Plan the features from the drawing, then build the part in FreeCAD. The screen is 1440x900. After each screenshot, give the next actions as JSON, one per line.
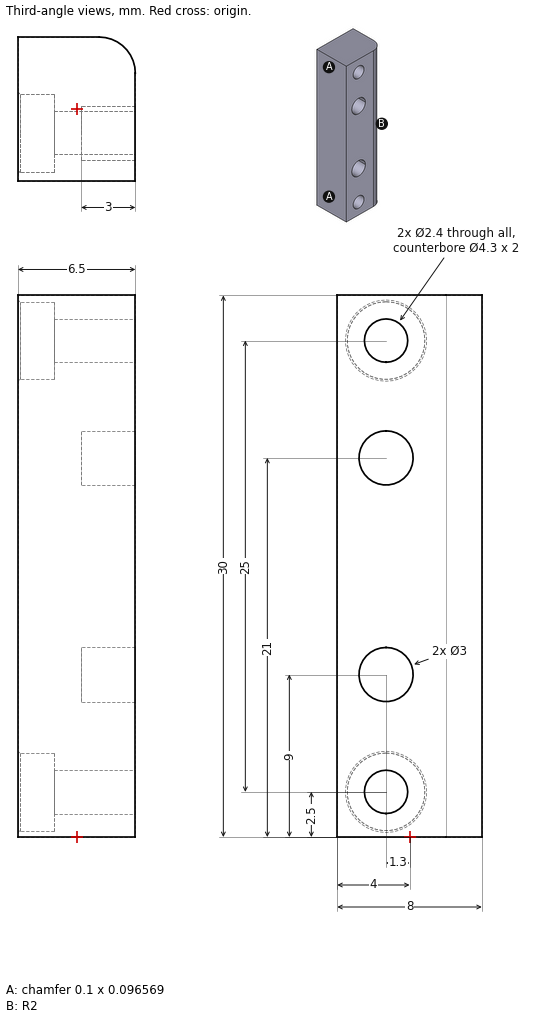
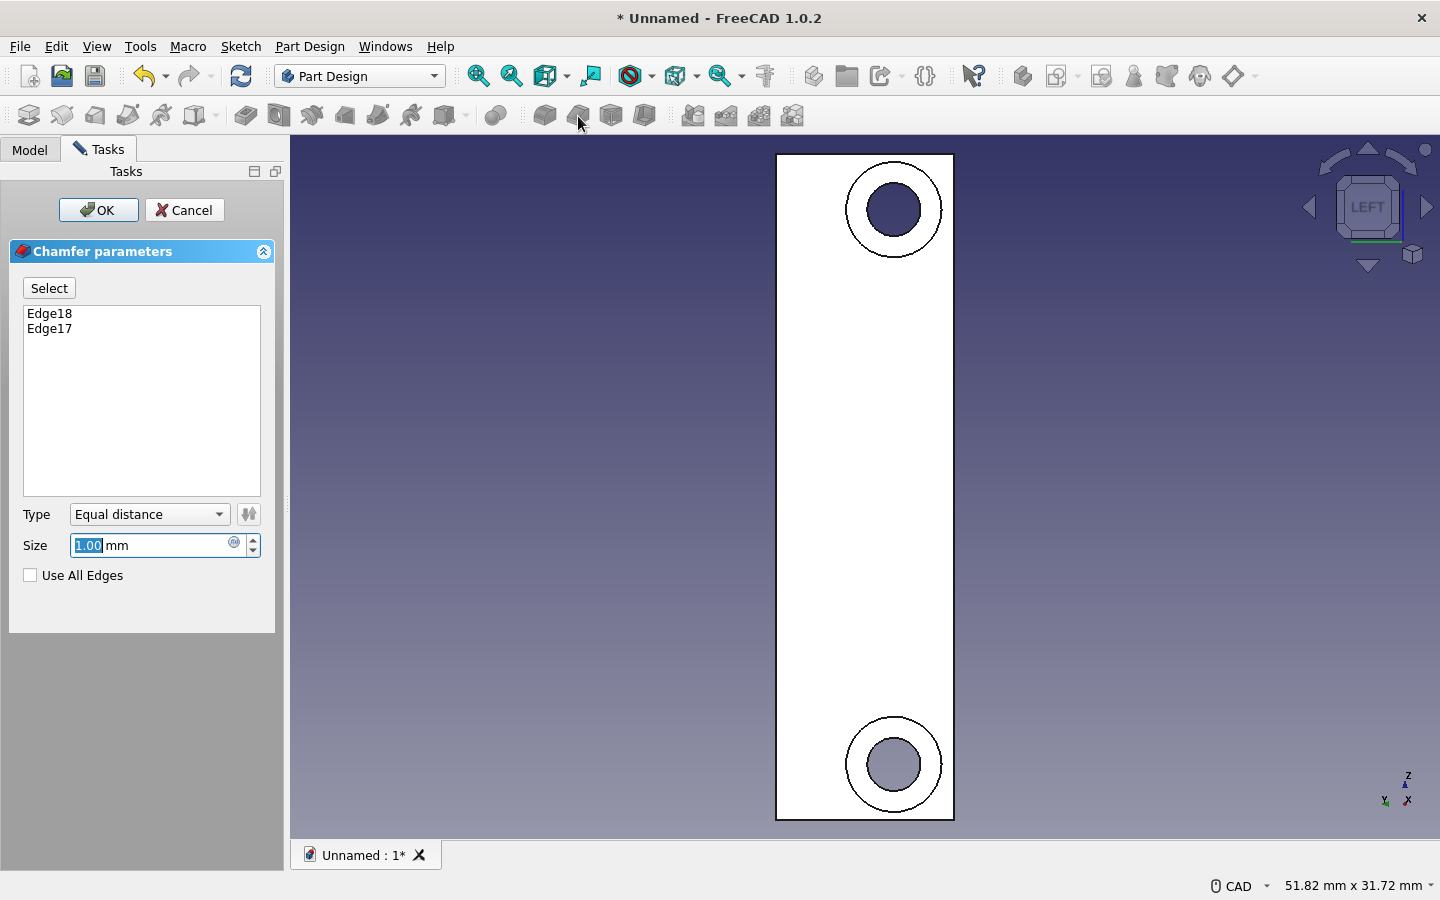
{"action": "type", "text": "0.1"}
{"action": "key", "text": "Tab"}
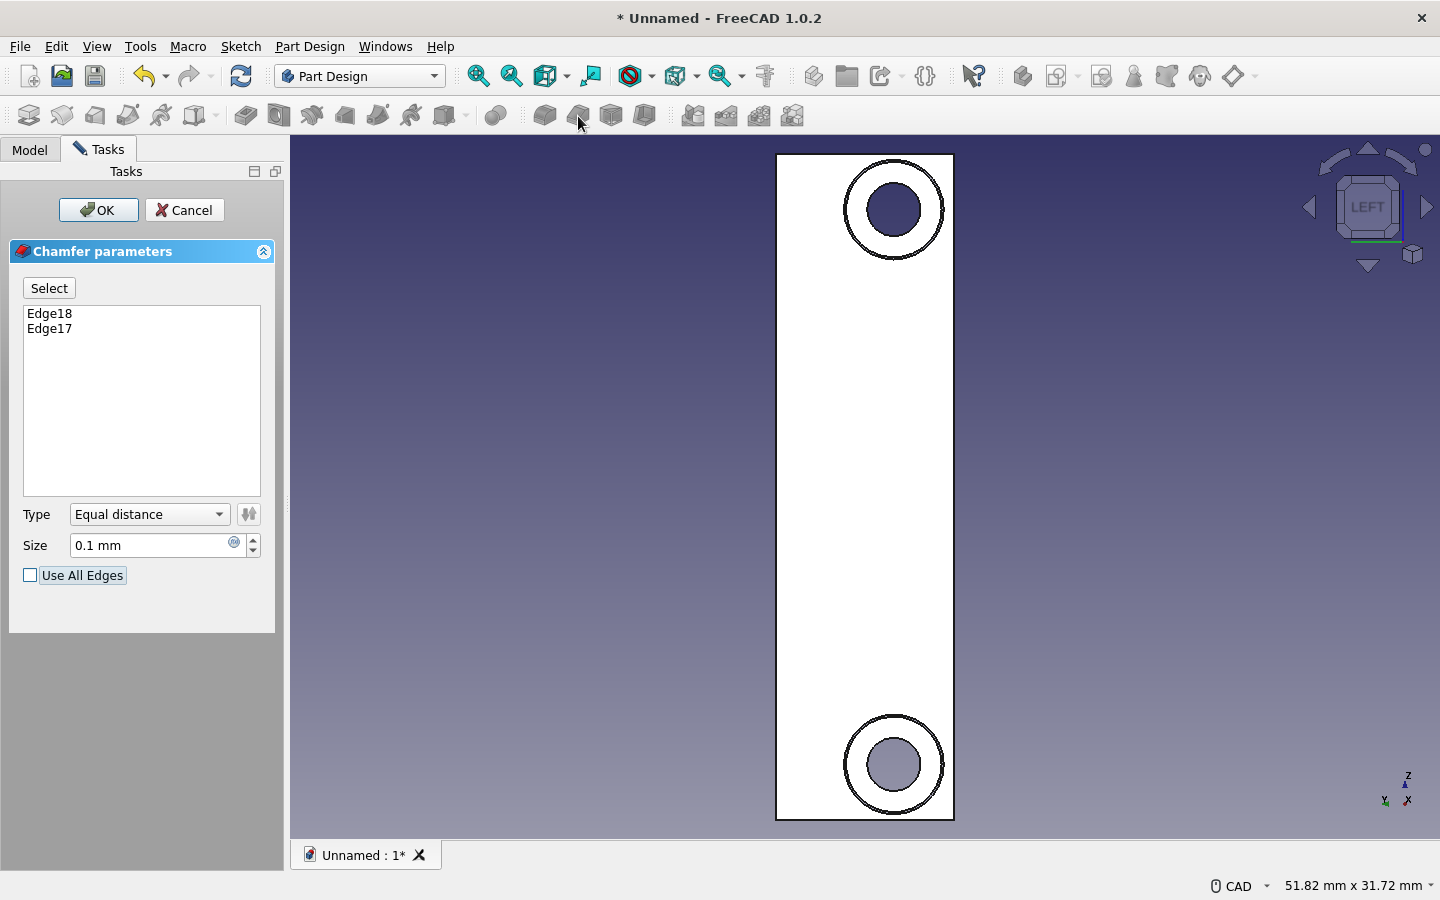
{"action": "left_click", "coordinate": [150, 514]}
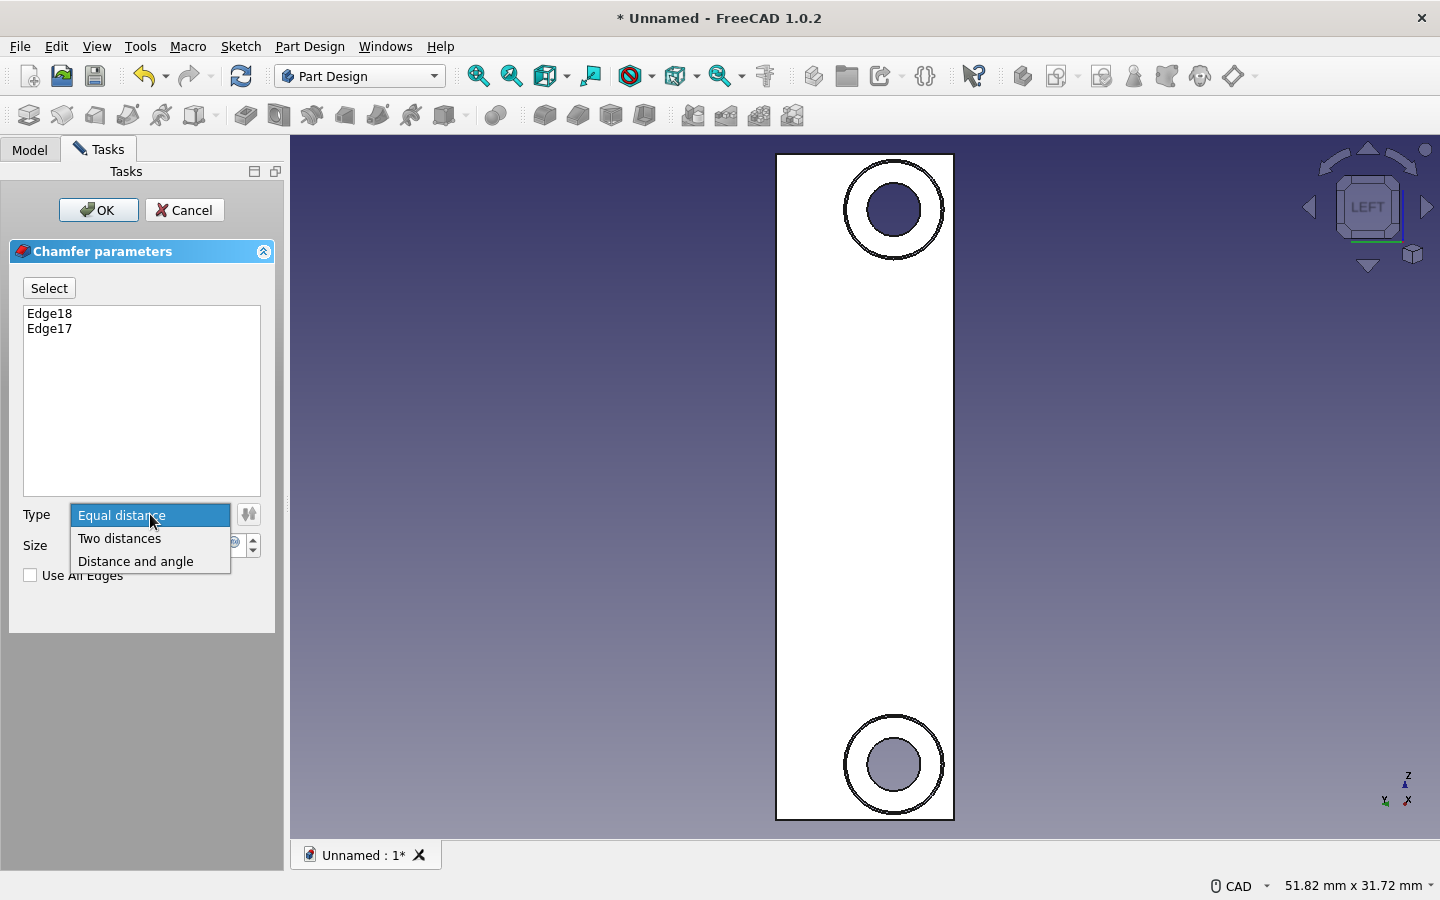
{"action": "left_click", "coordinate": [148, 538]}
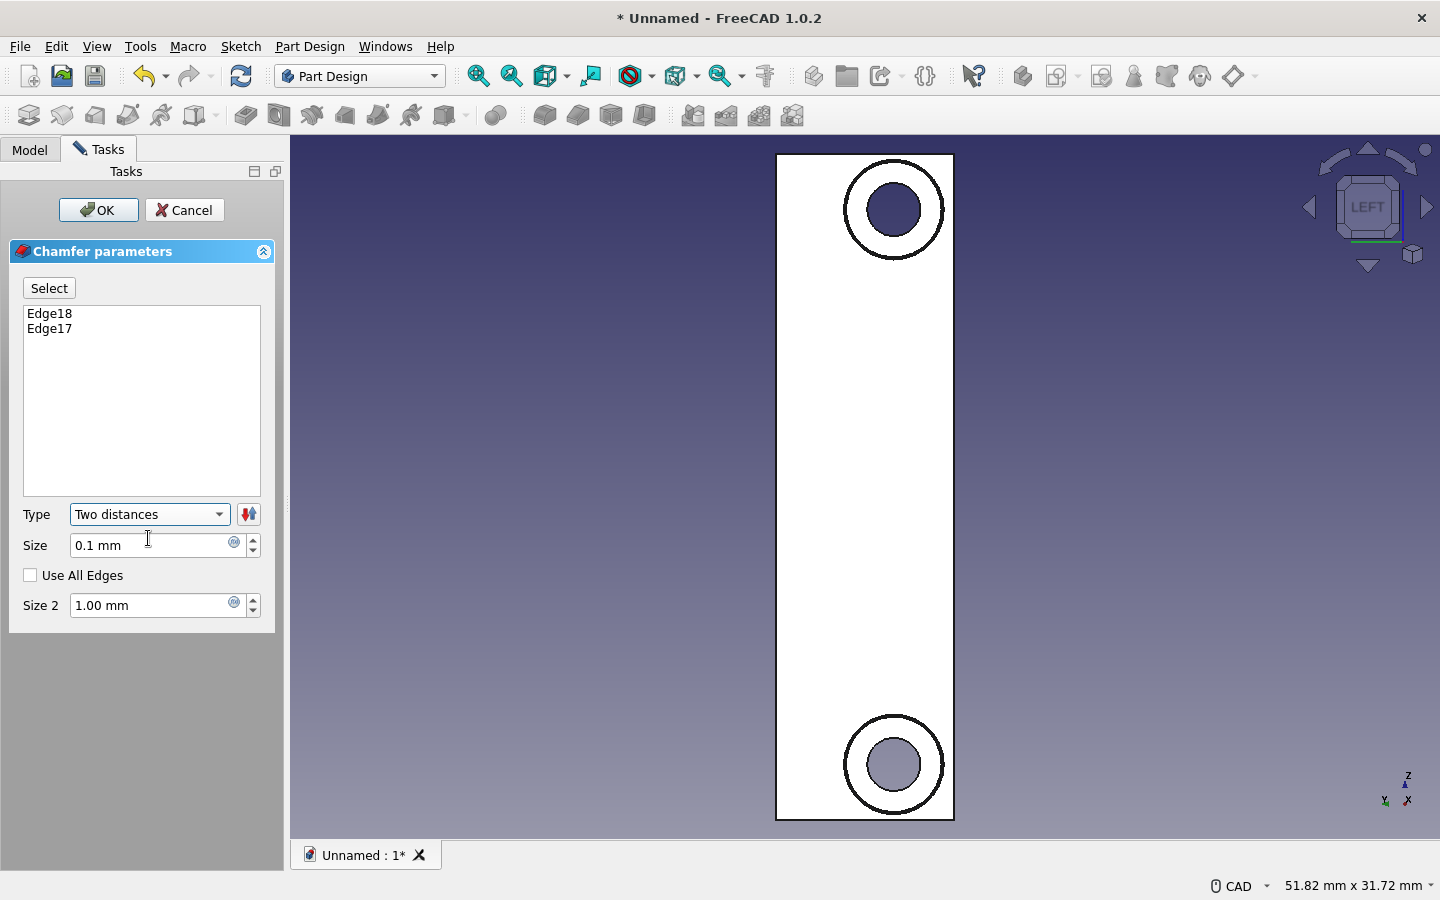
{"action": "triple_click", "coordinate": [158, 606]}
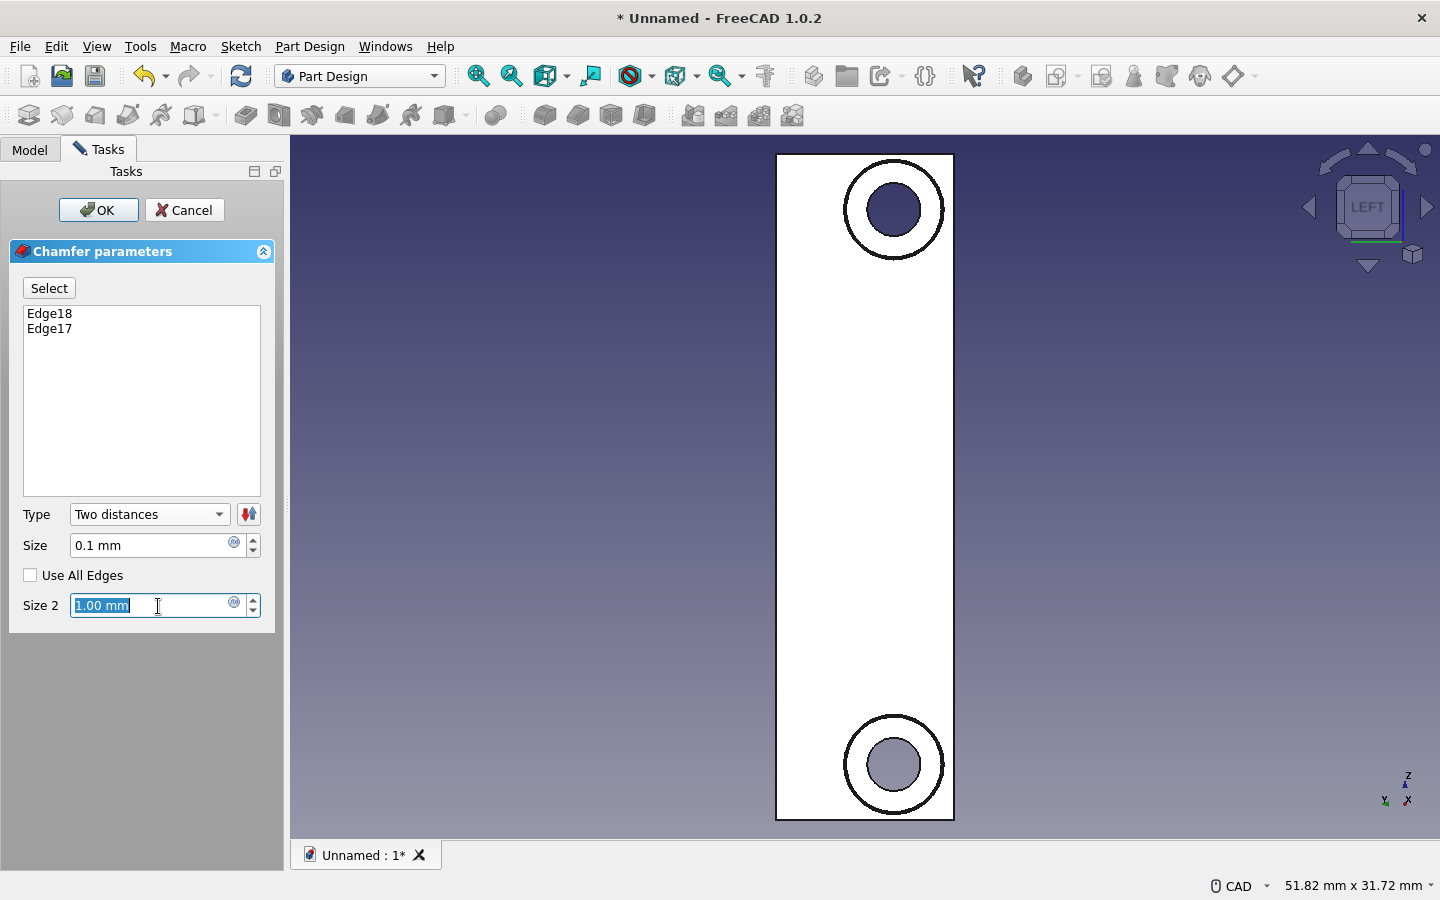
{"action": "type", "text": "0.096569"}
{"action": "key", "text": "Tab"}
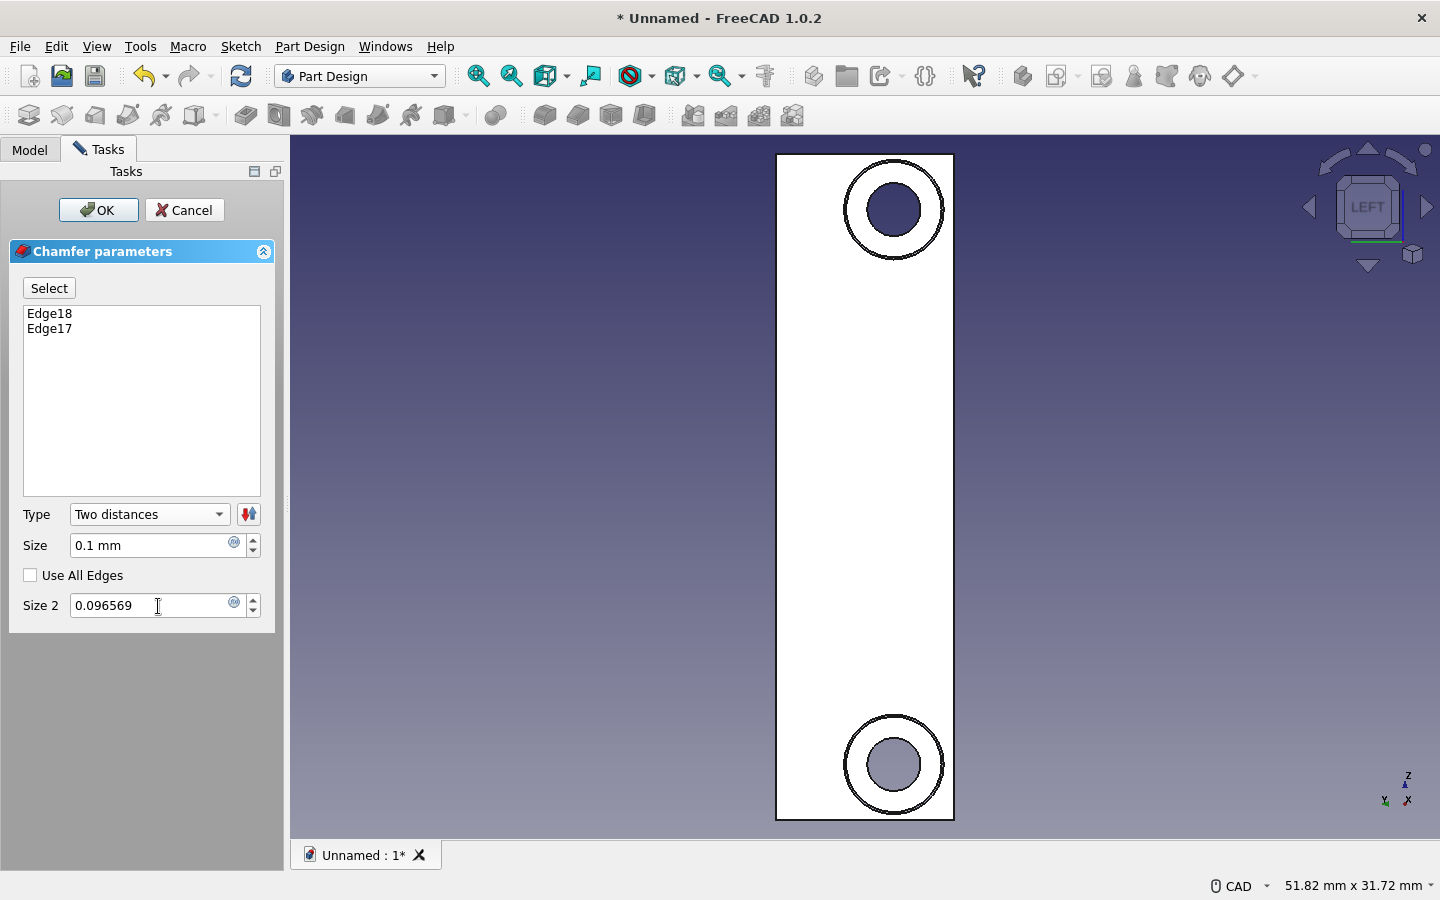
{"action": "left_click", "coordinate": [99, 210]}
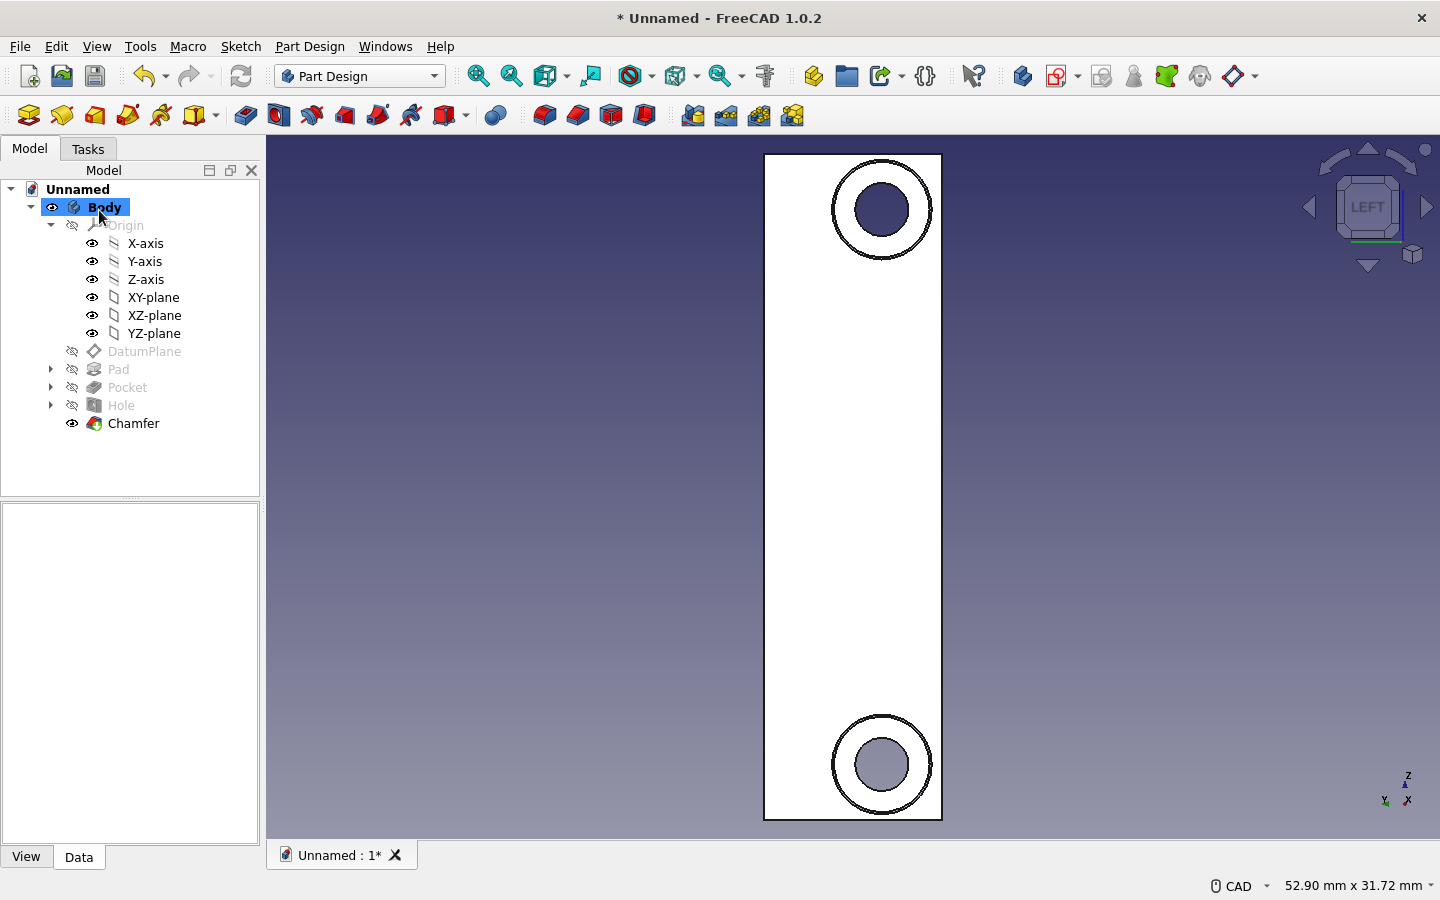
{"action": "key", "text": "0"}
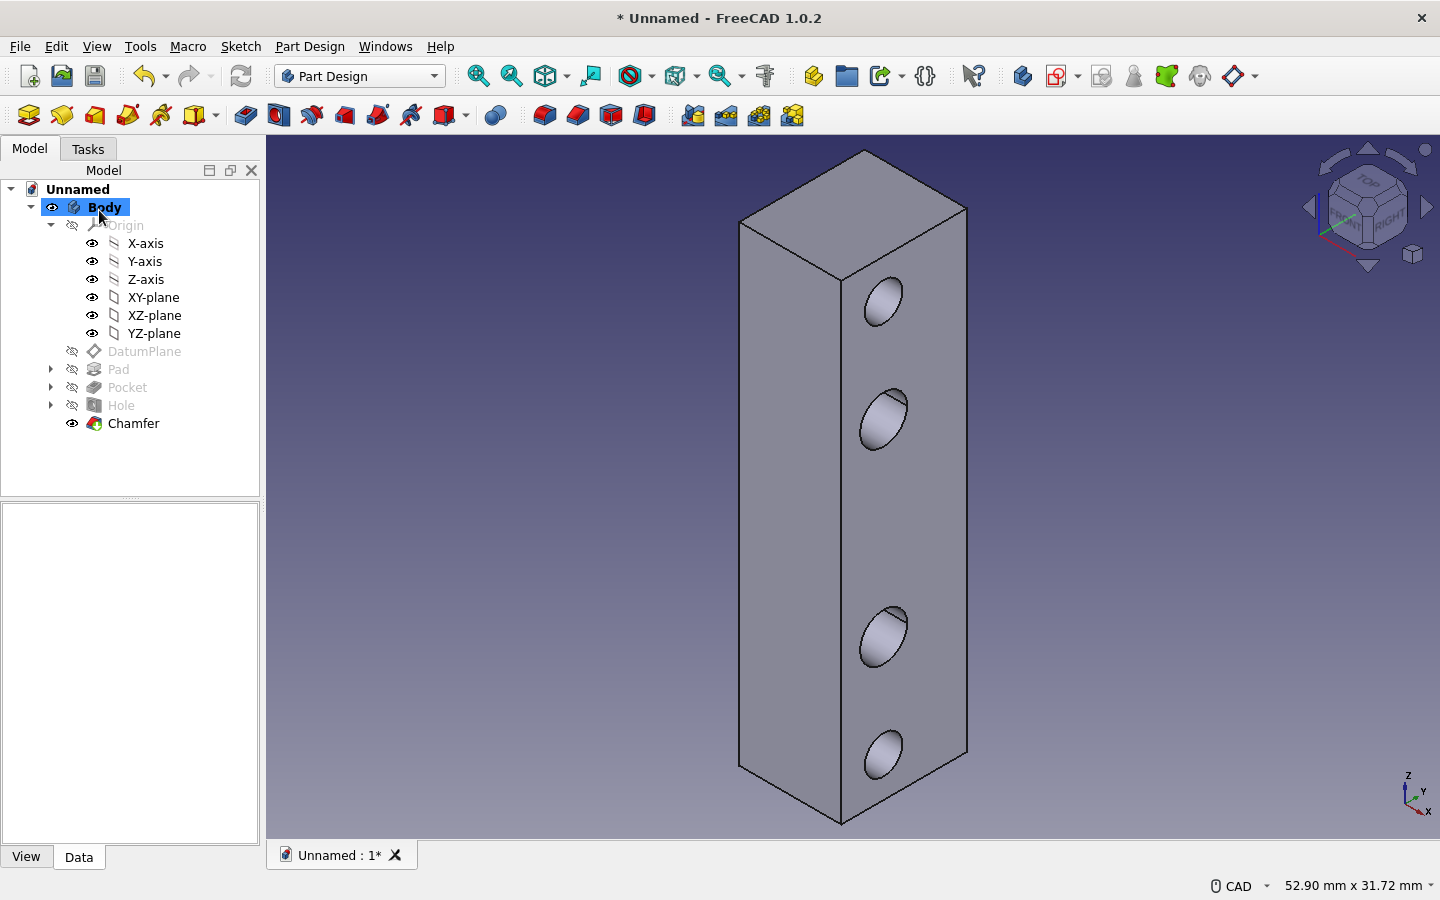
{"action": "key", "text": "2"}